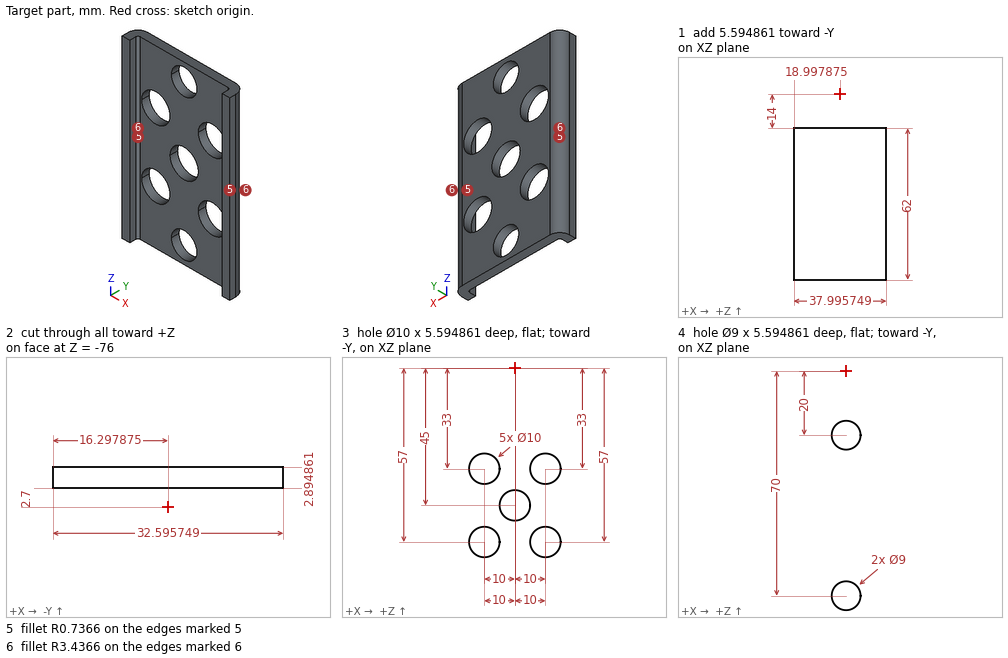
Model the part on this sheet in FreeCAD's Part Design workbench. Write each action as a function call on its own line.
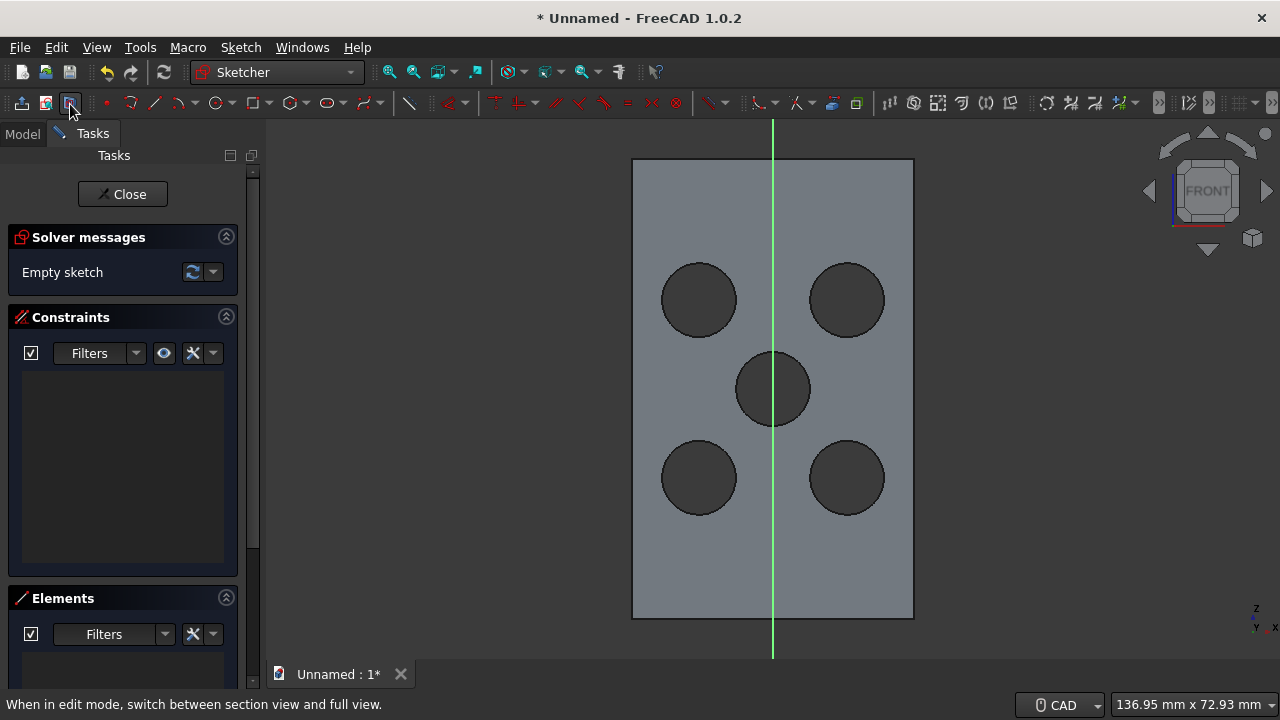
scroll(565, 506, down, 2)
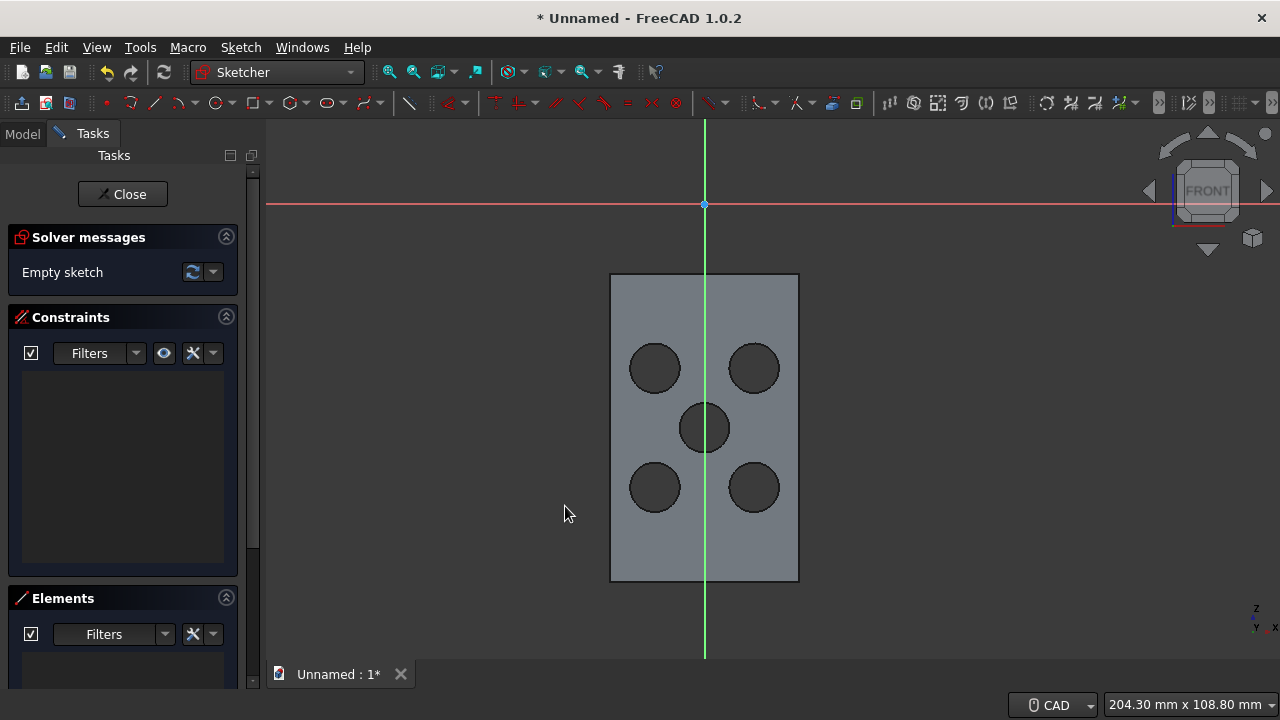
click(216, 104)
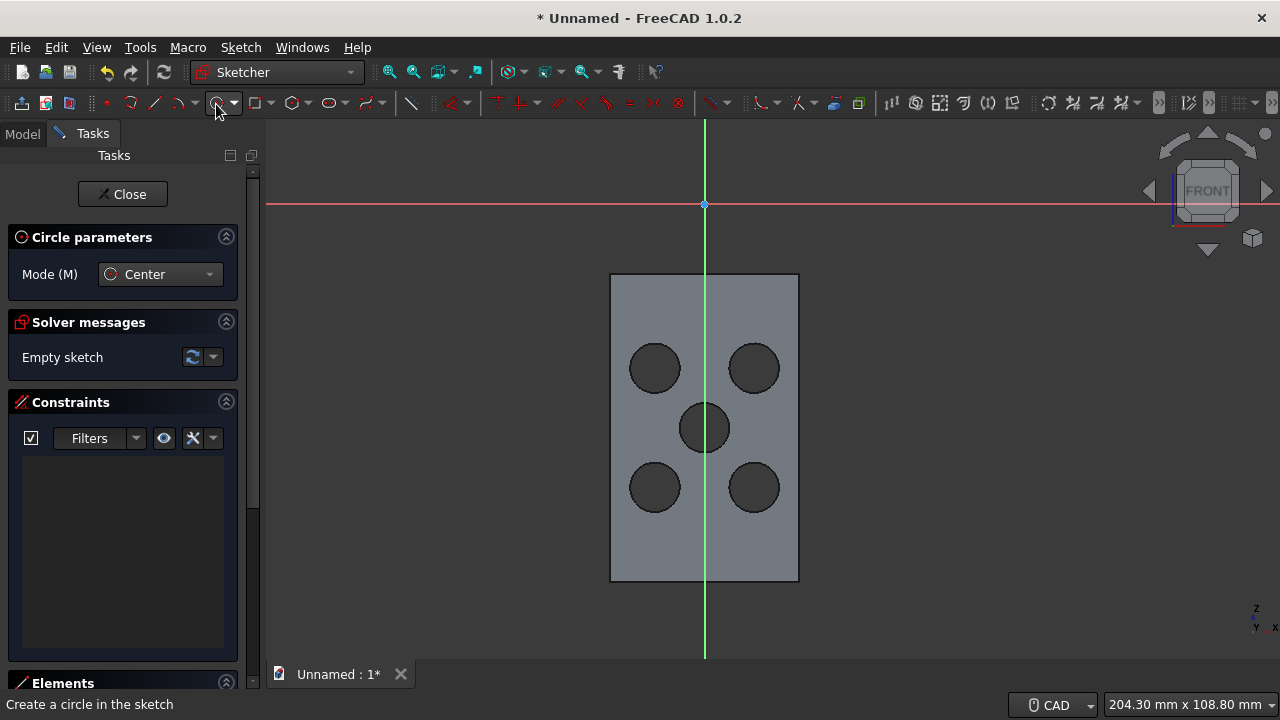
click(705, 552)
move(720, 536)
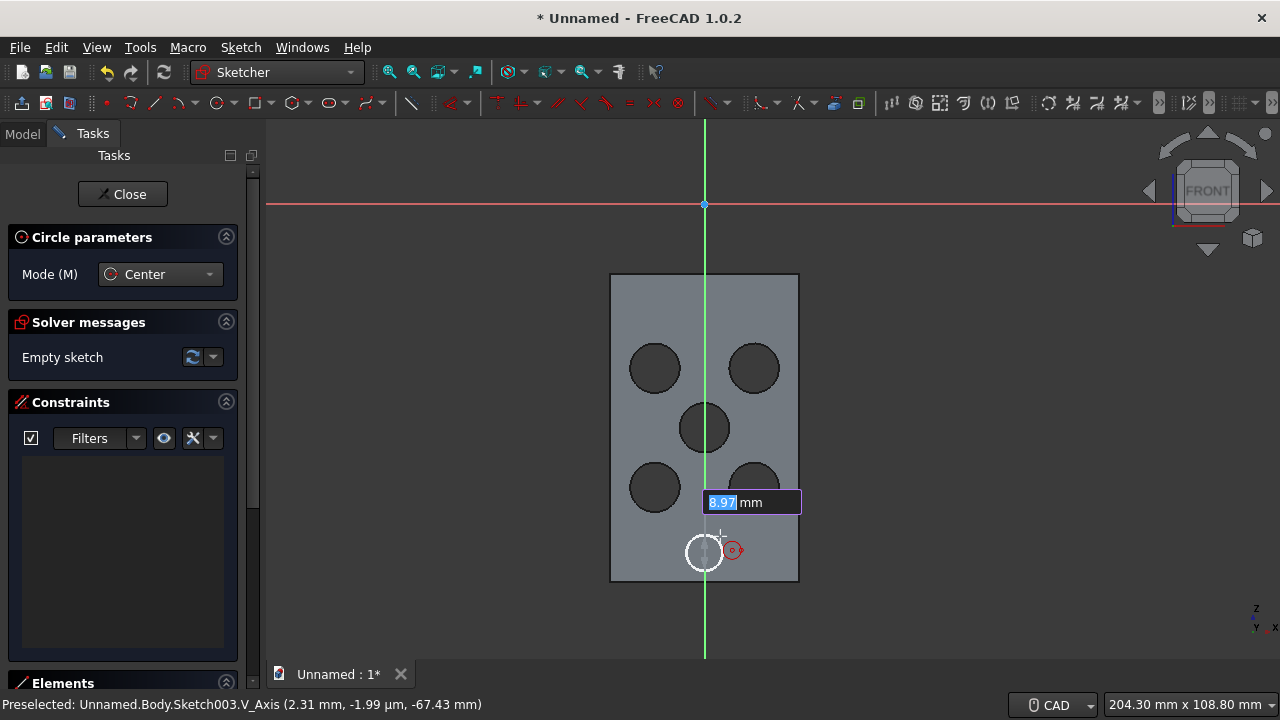
text(9)
key(Return)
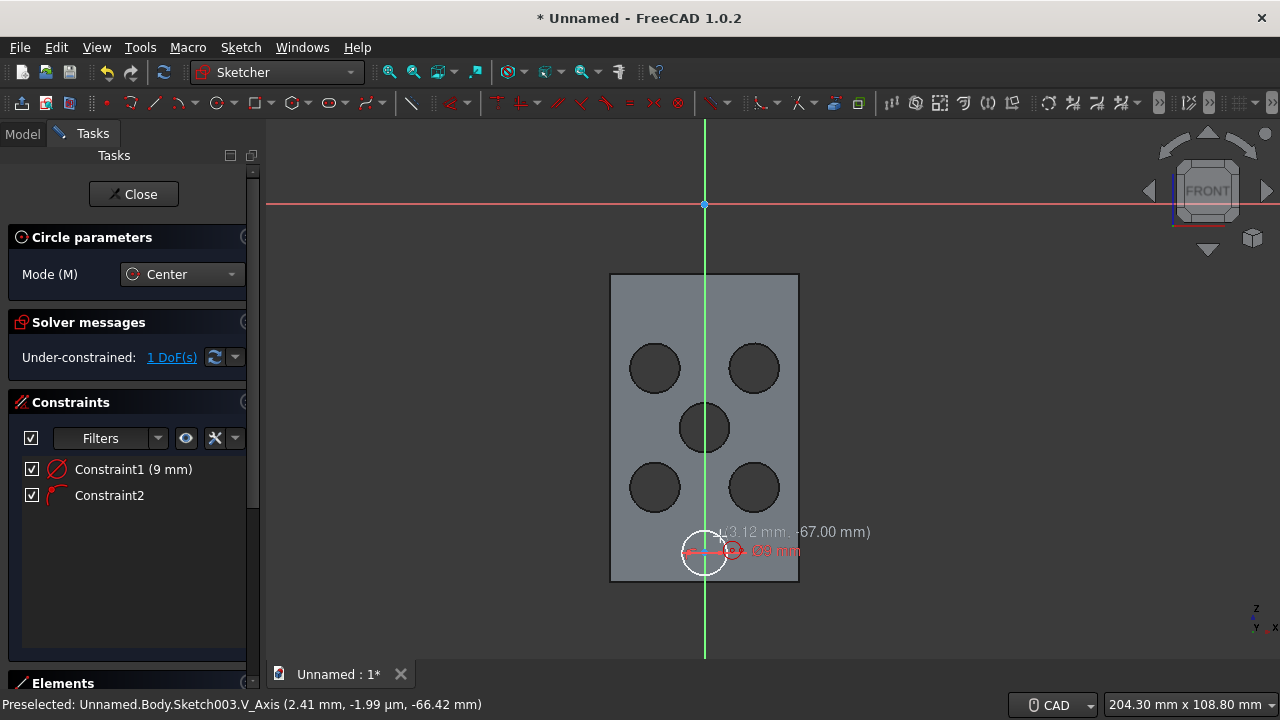
click(705, 304)
move(720, 288)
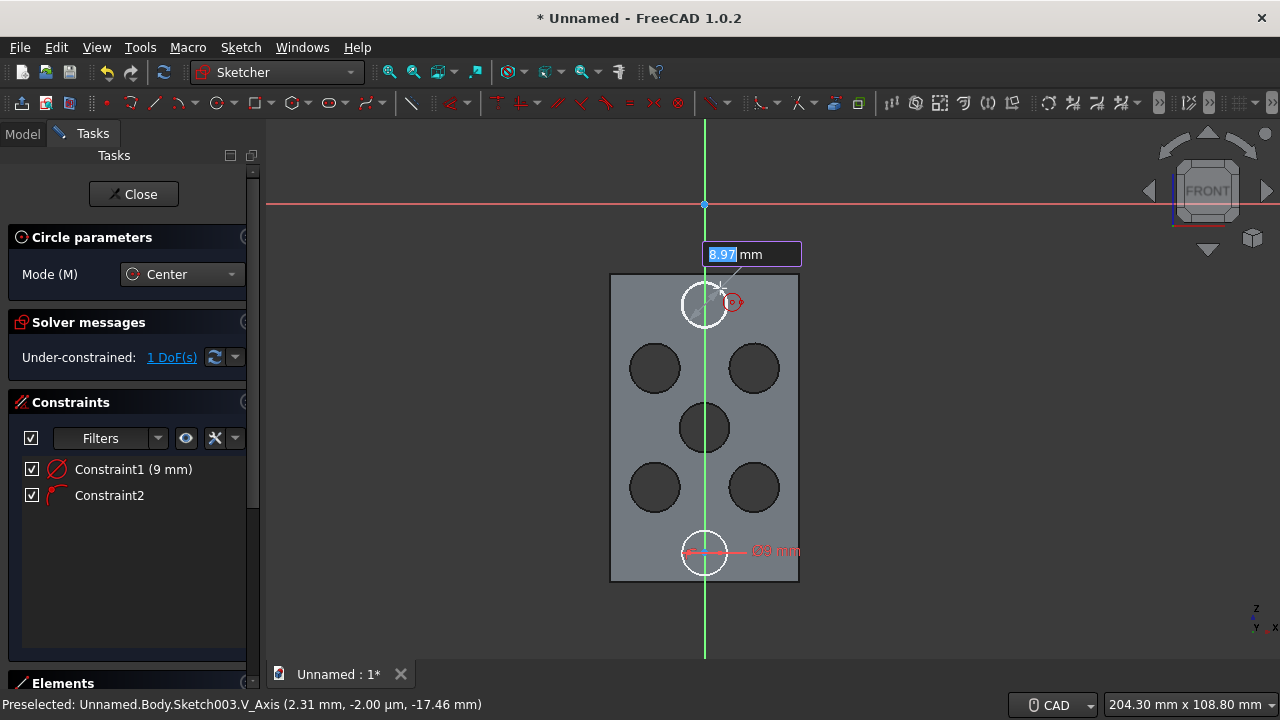
text(9)
key(Return)
key(Escape)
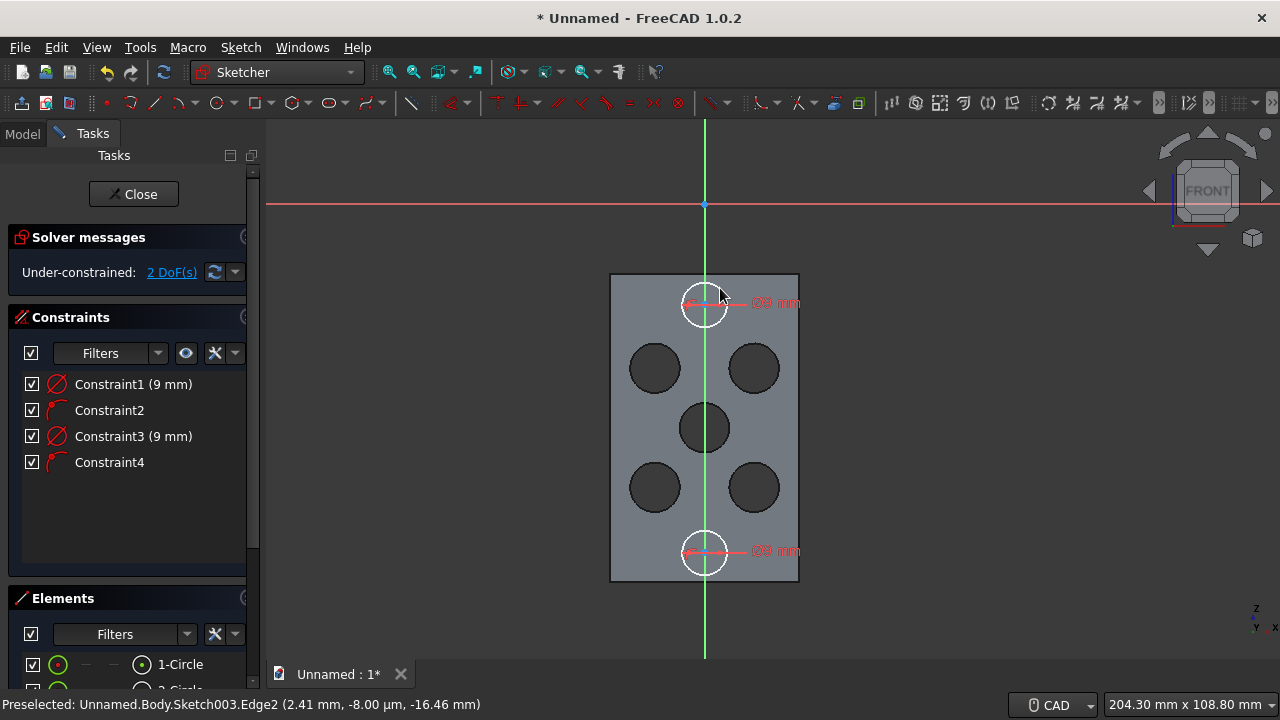
key(d)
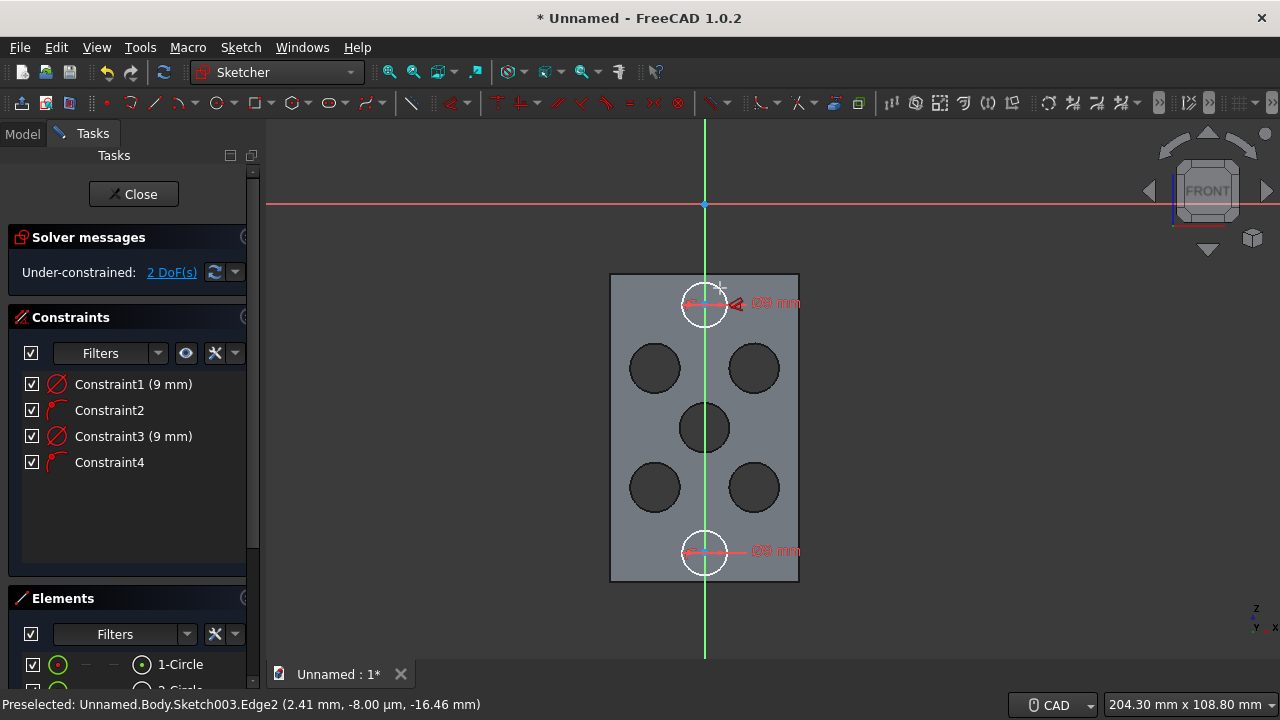
click(705, 553)
click(739, 379)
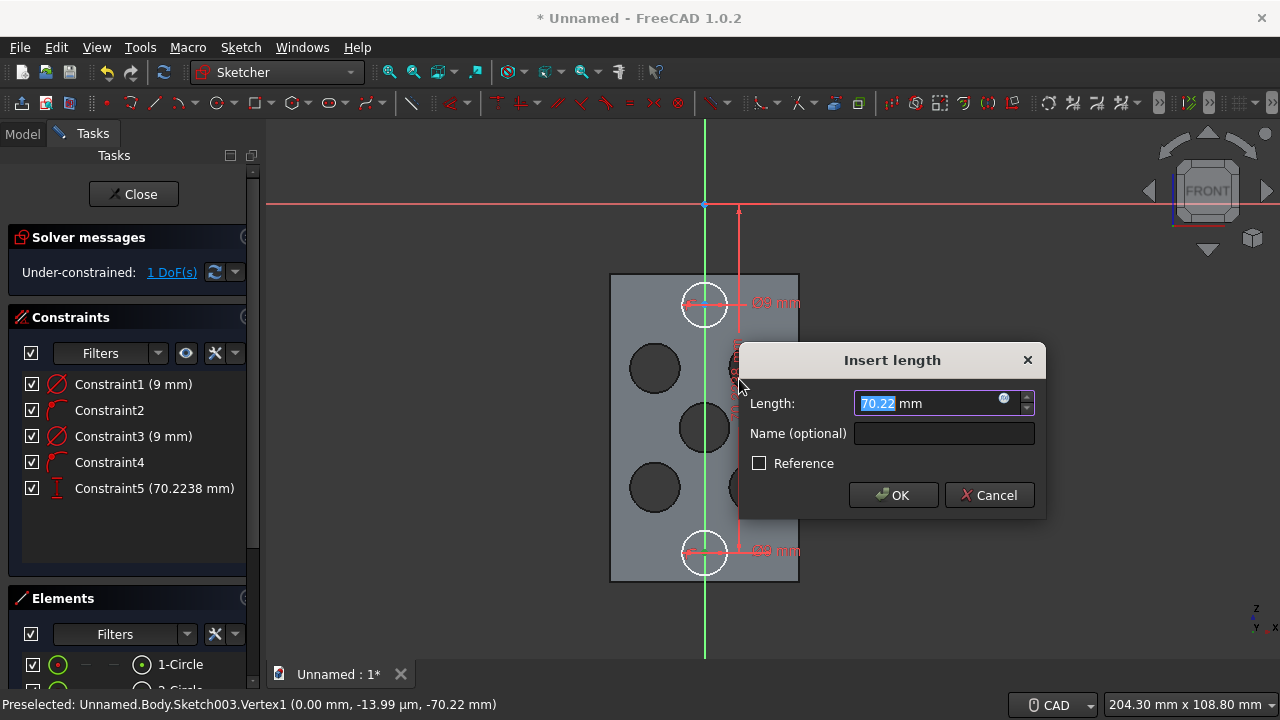
text(70)
key(Return)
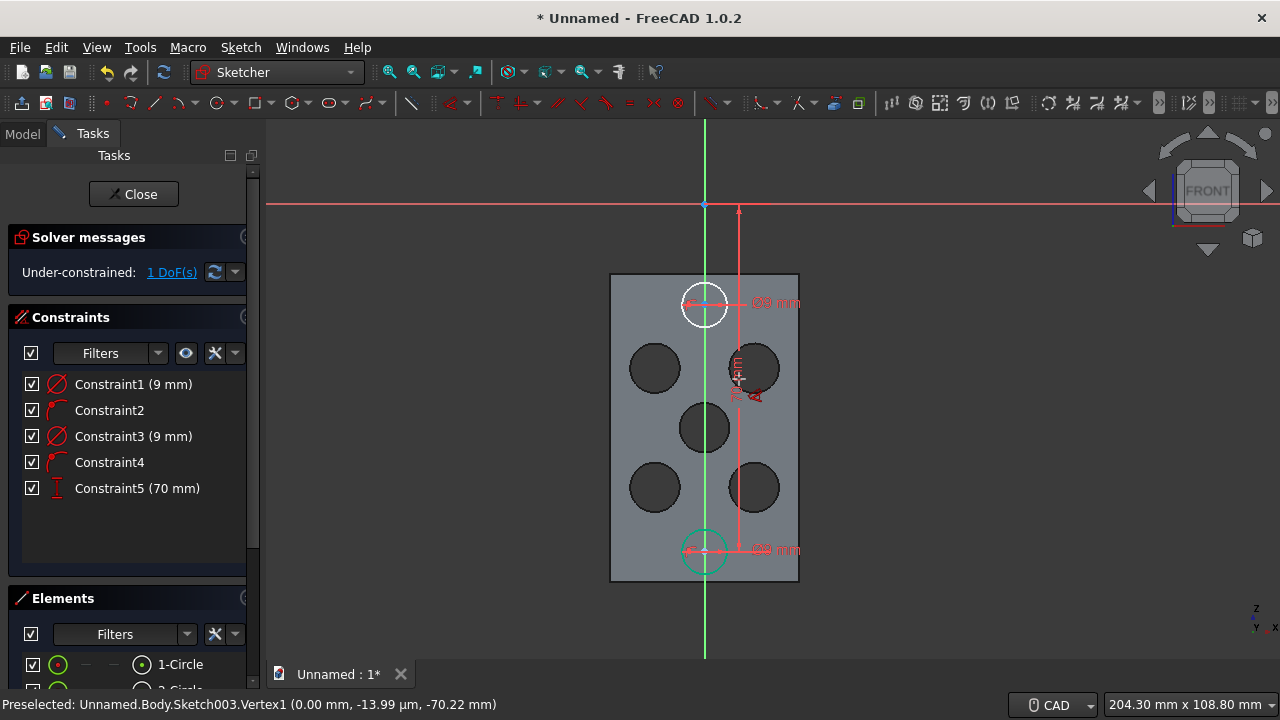
click(705, 305)
click(739, 255)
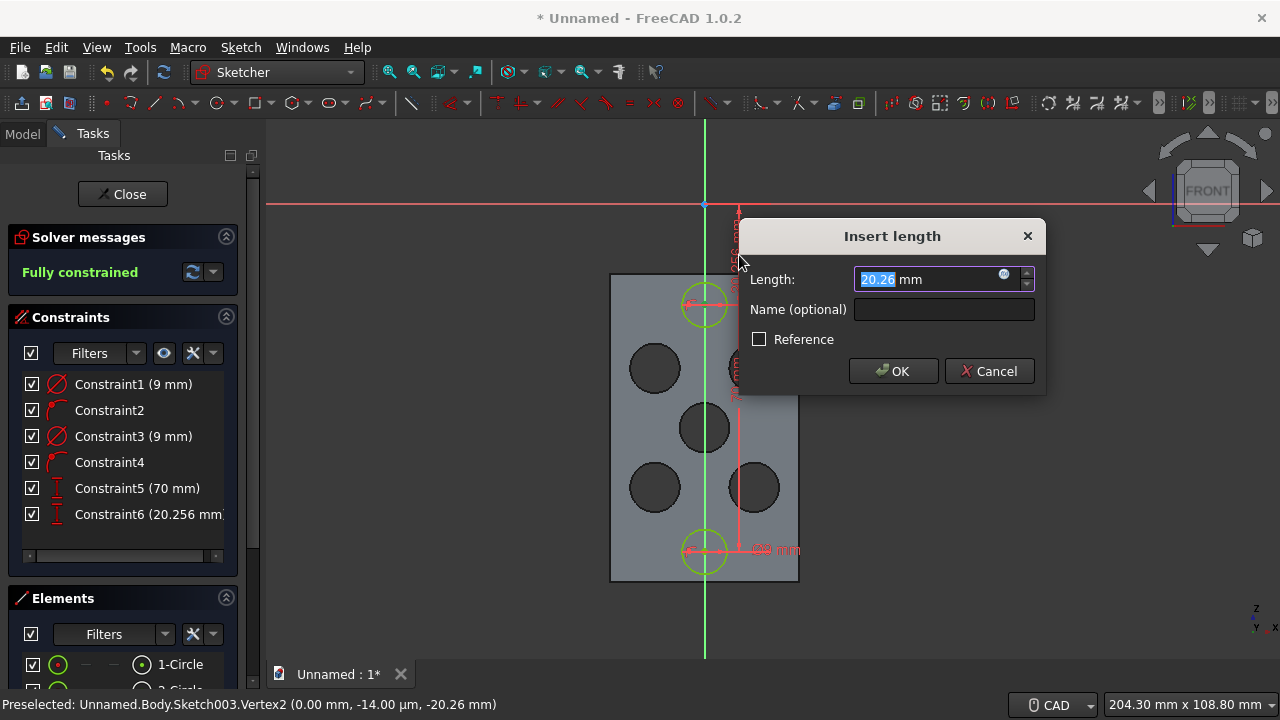
text(20)
key(Return)
key(Escape)